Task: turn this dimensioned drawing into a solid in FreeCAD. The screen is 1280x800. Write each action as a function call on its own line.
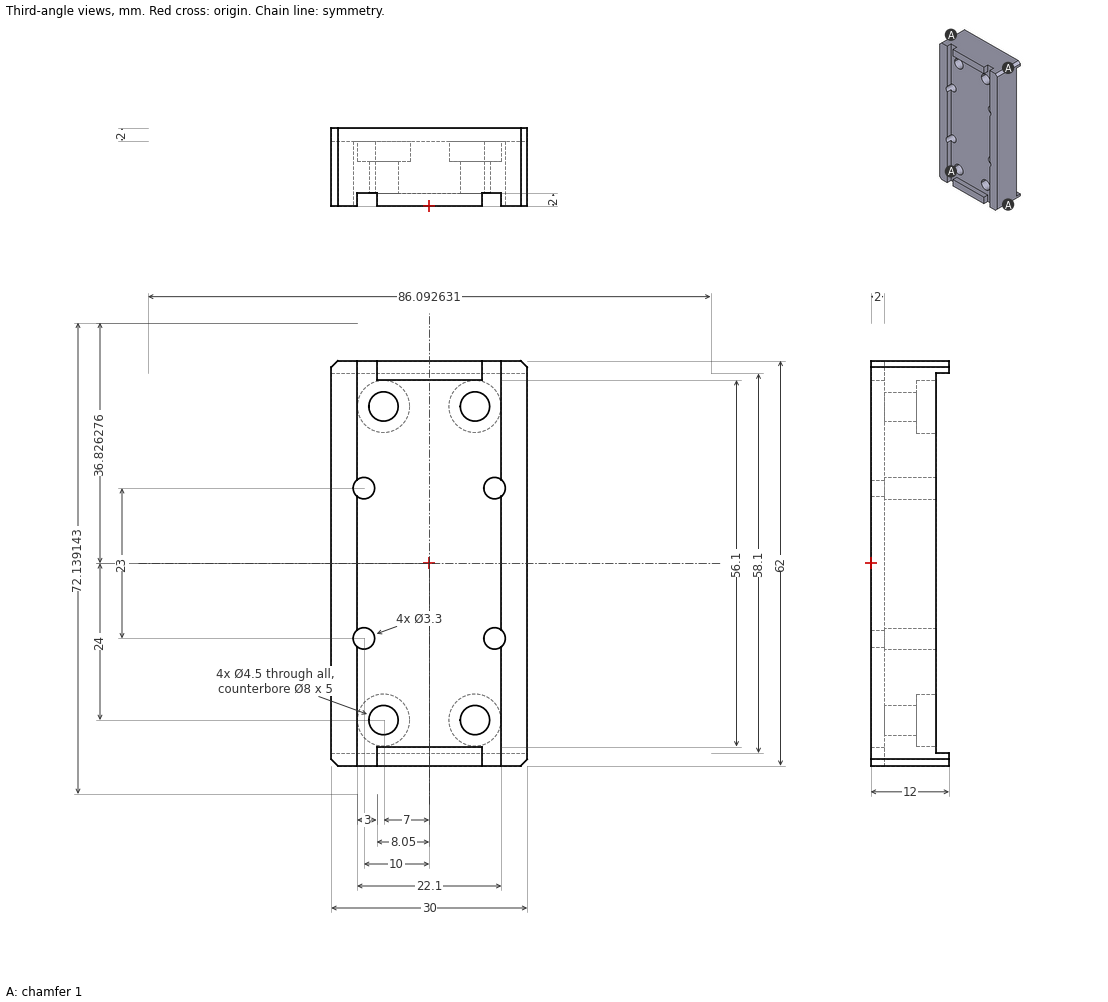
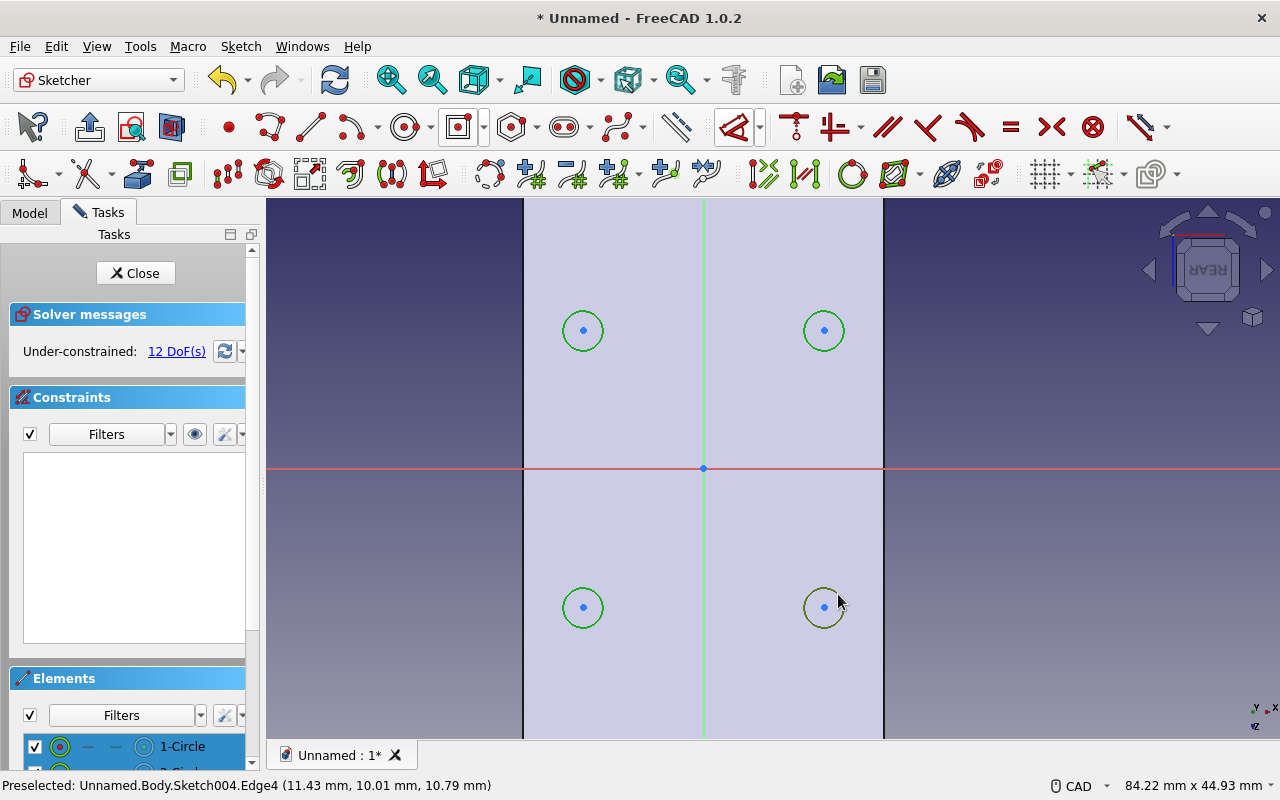
click(1011, 128)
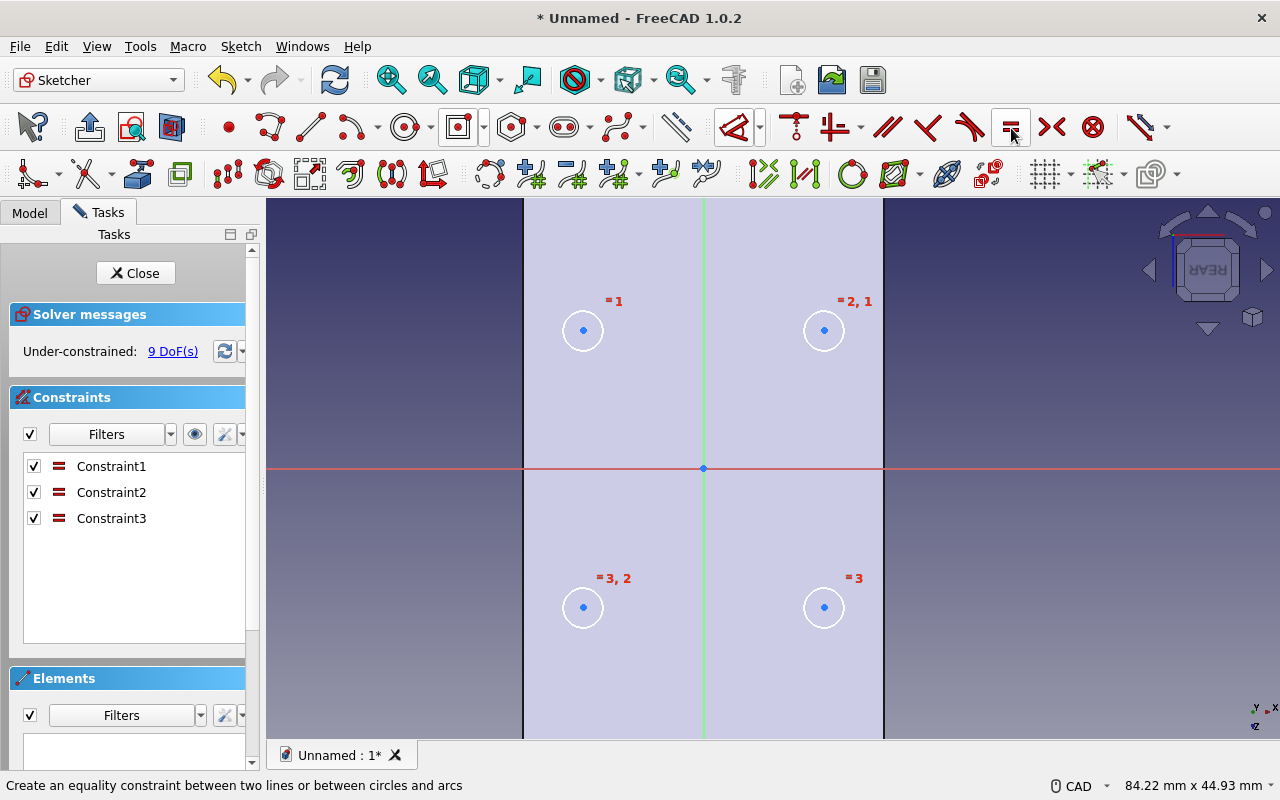
click(583, 331)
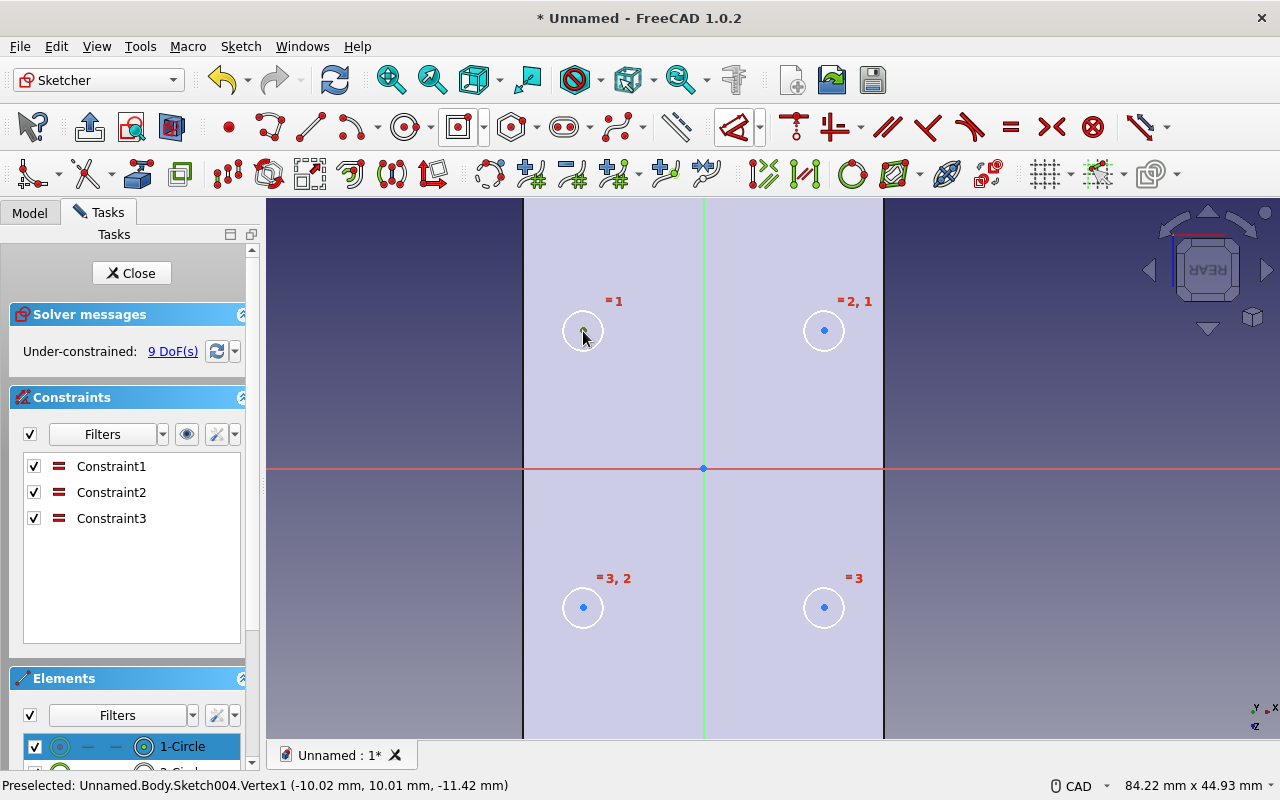
click(824, 331)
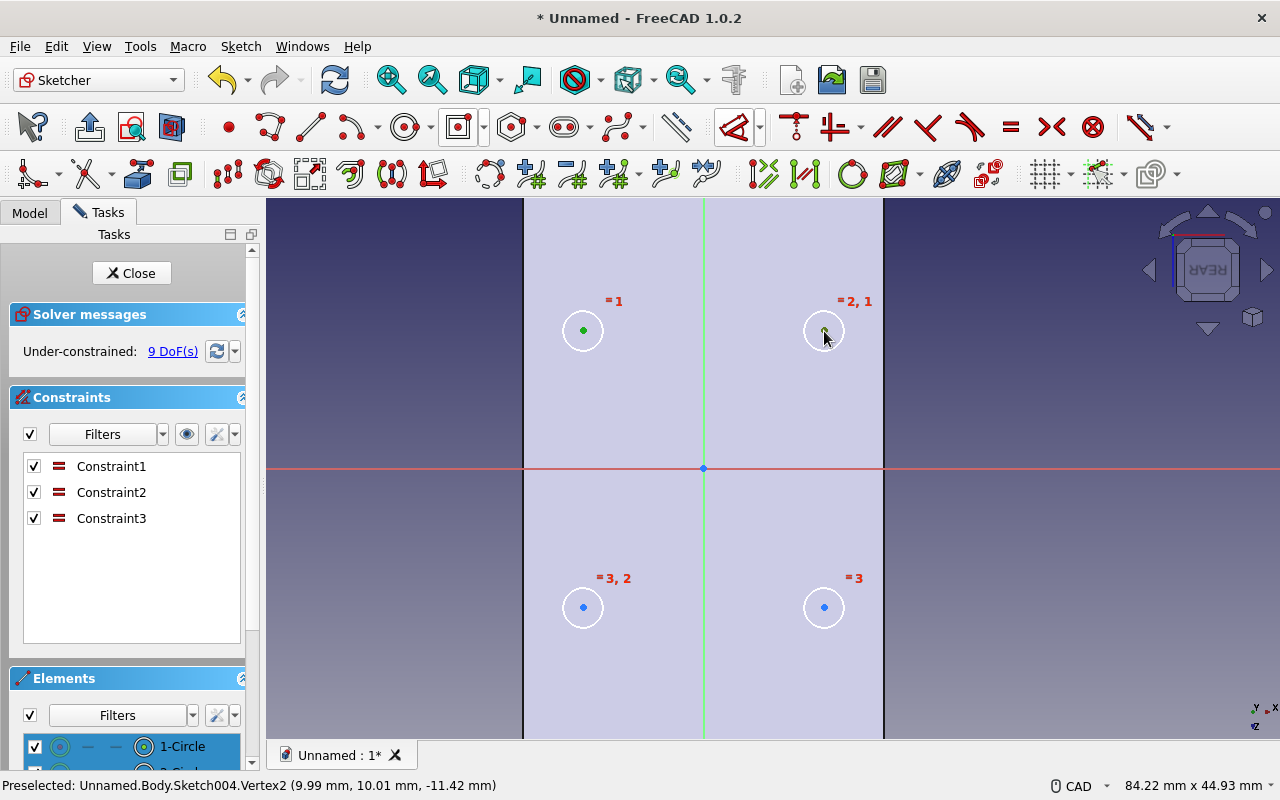
click(704, 676)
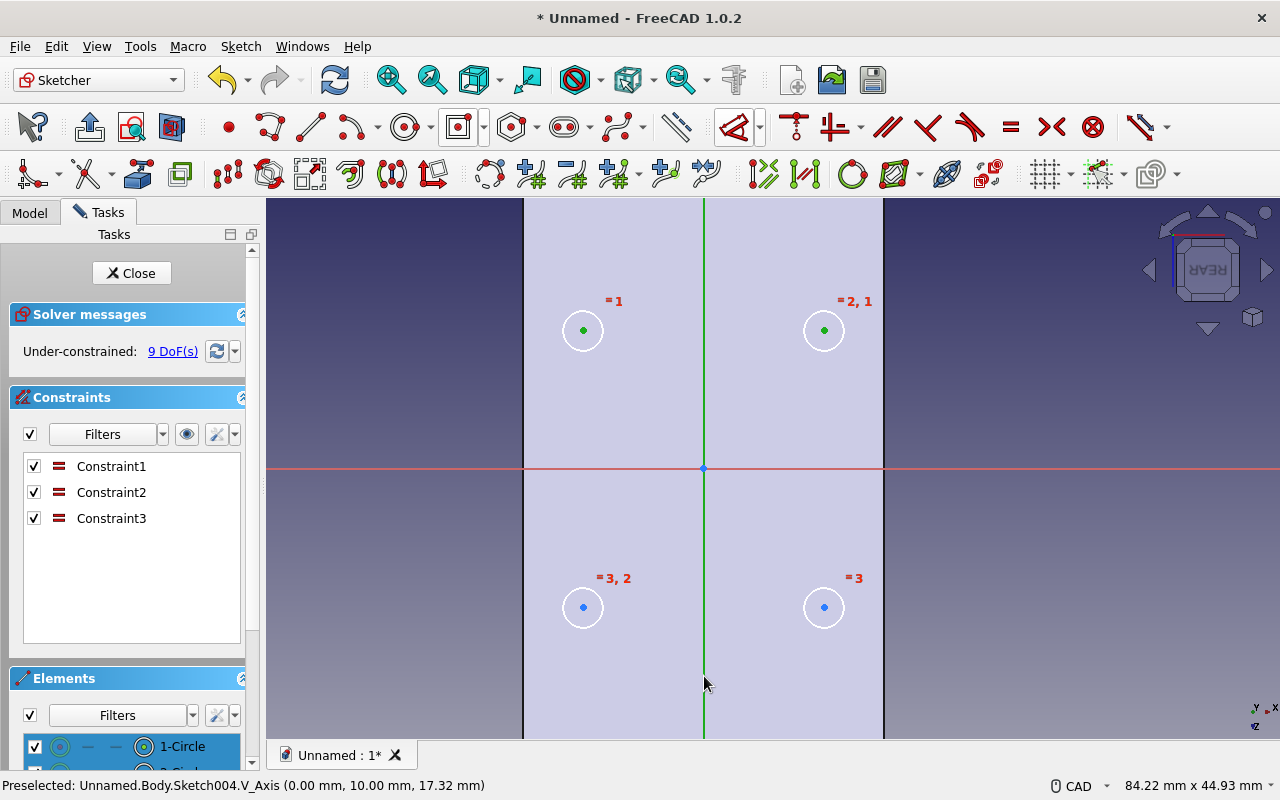
click(1052, 128)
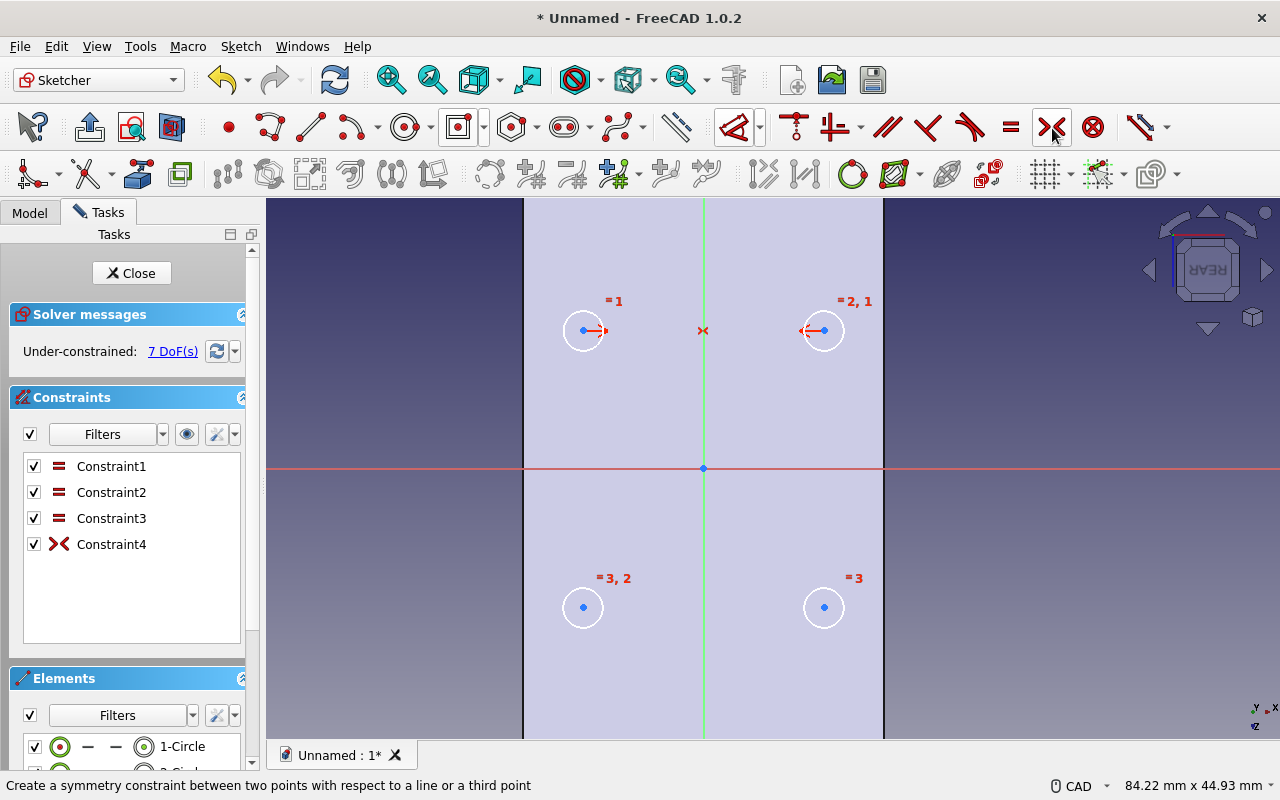
click(583, 331)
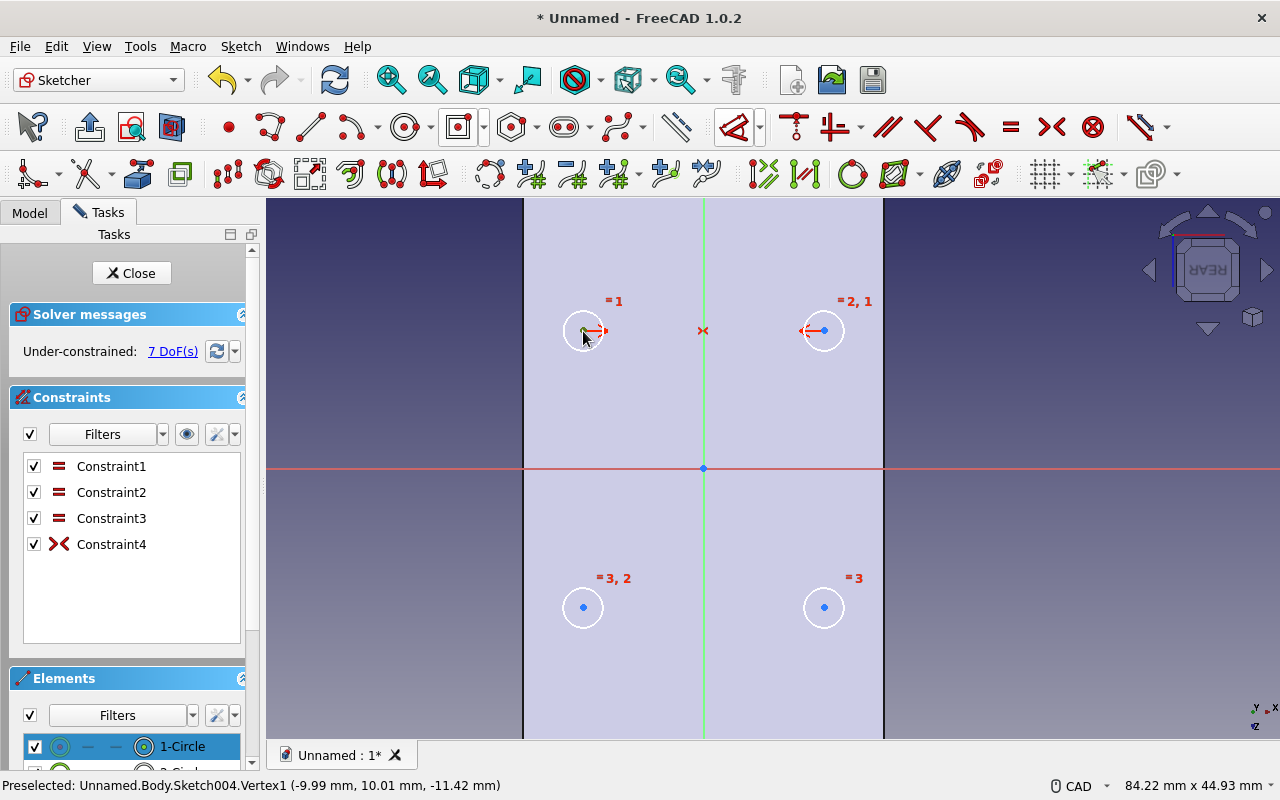
click(583, 608)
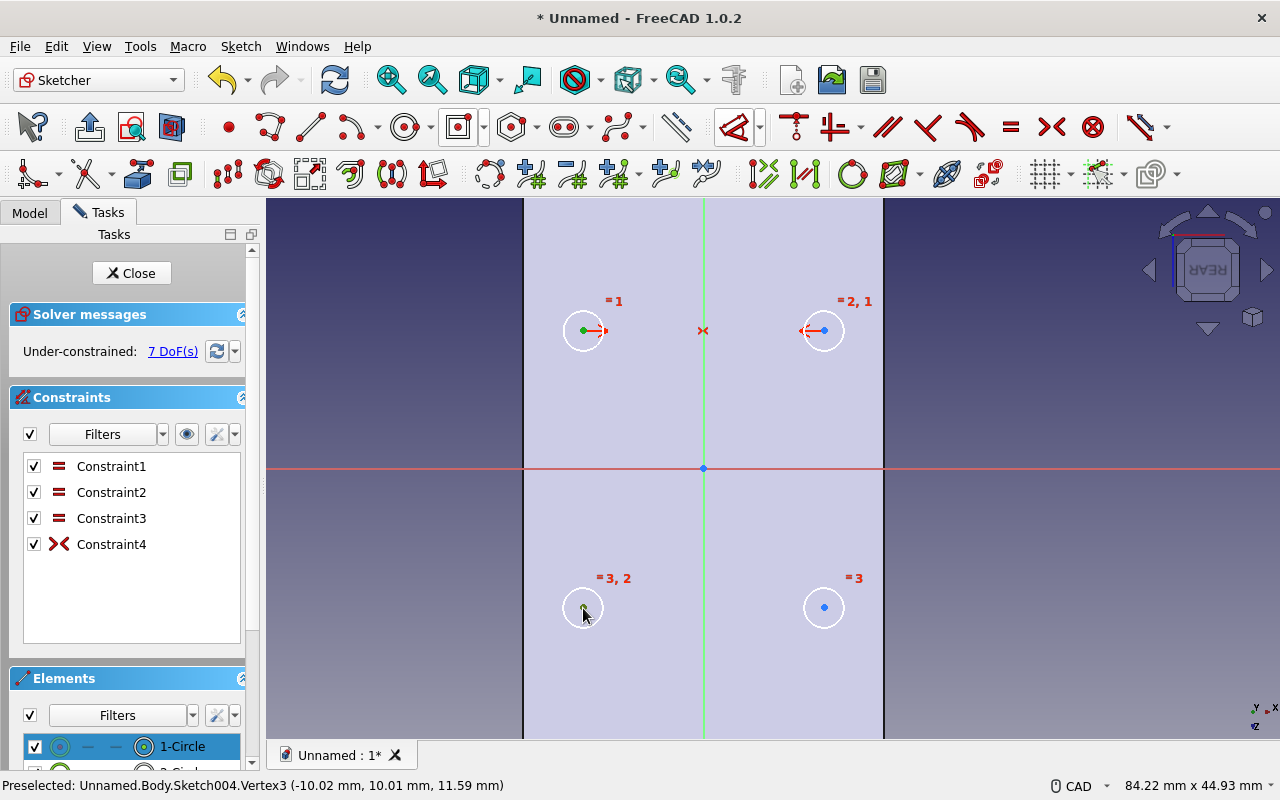
click(353, 468)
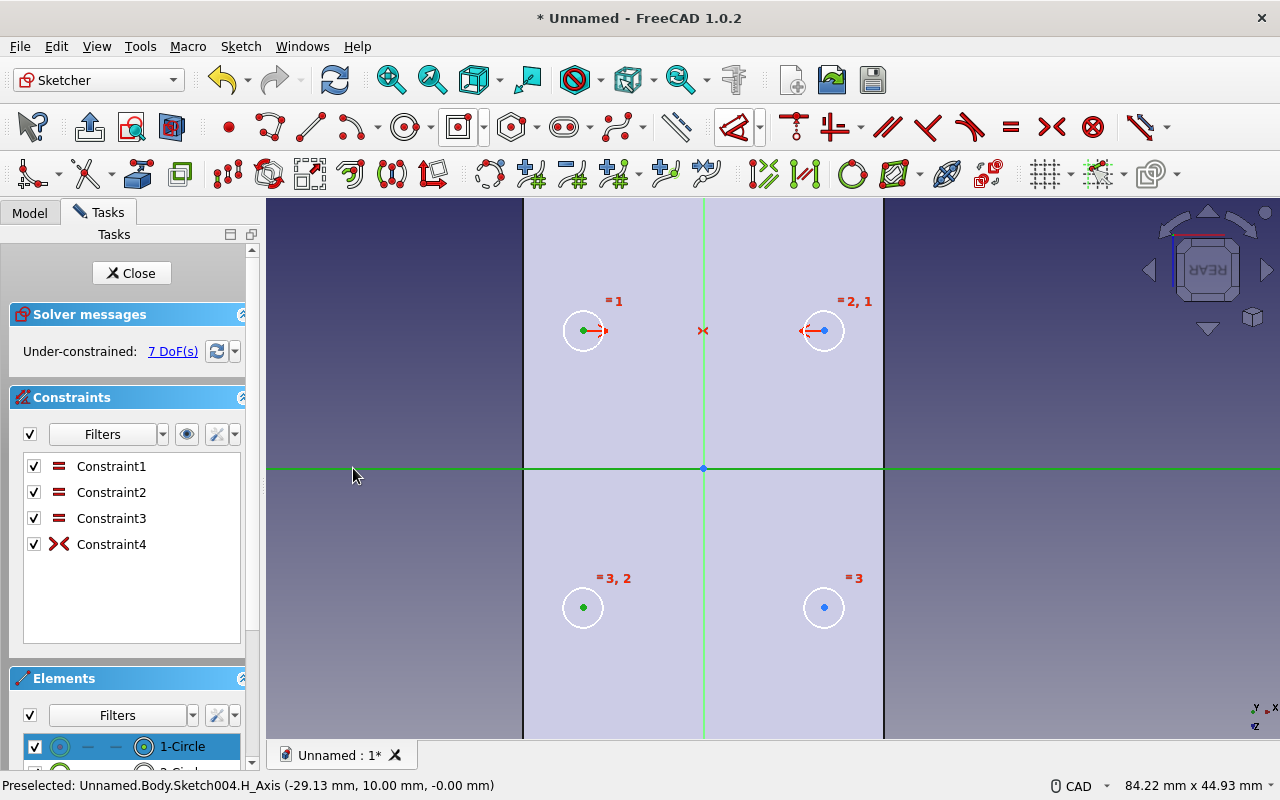
click(1052, 128)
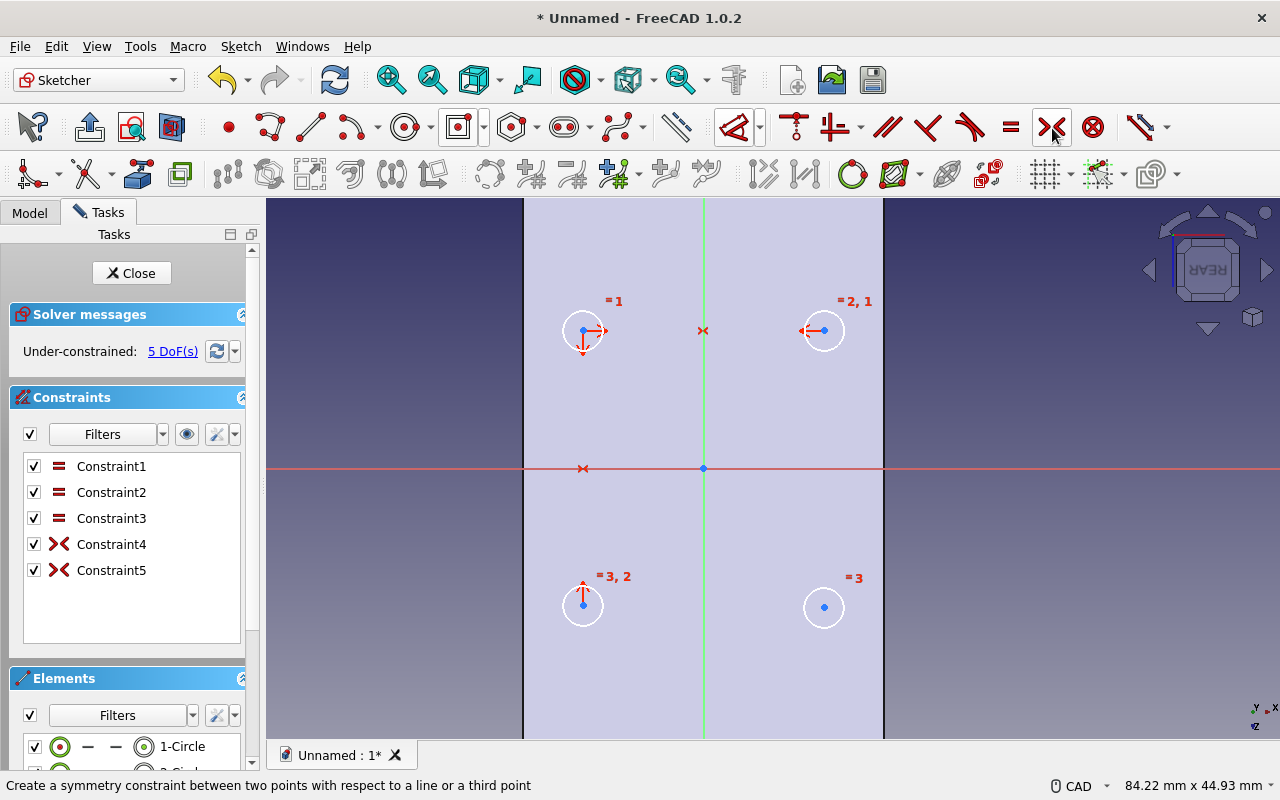
click(824, 331)